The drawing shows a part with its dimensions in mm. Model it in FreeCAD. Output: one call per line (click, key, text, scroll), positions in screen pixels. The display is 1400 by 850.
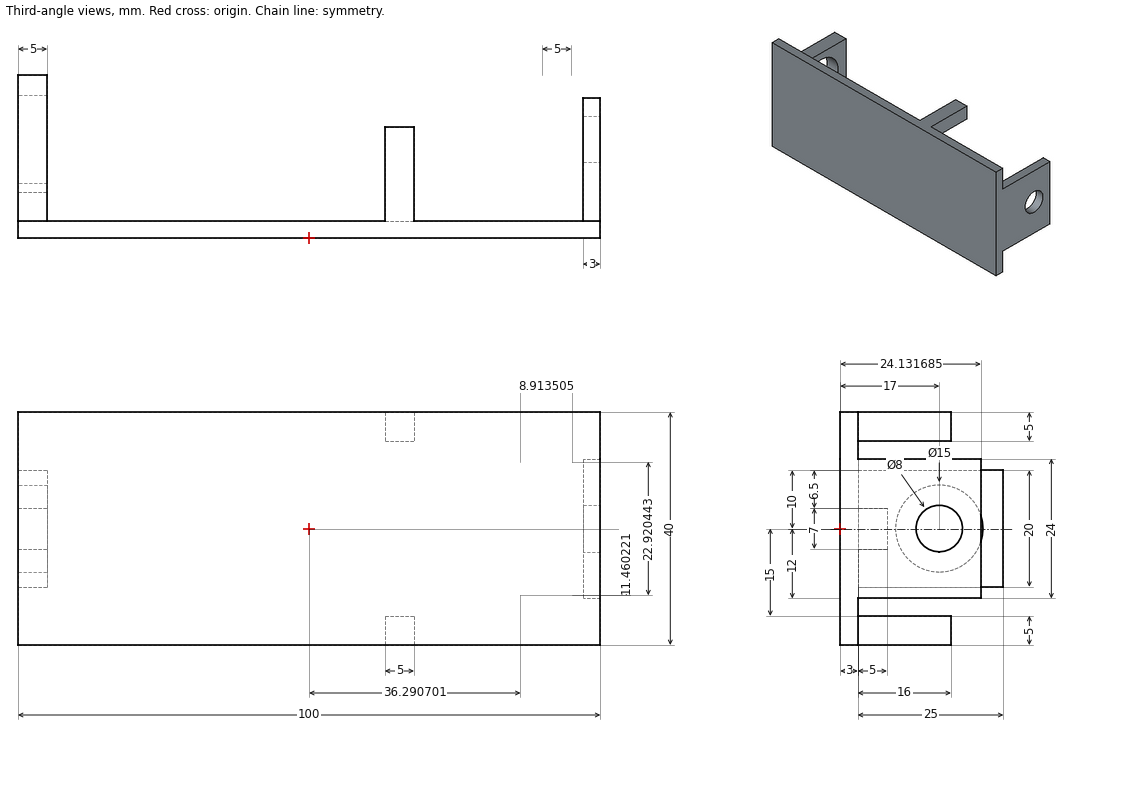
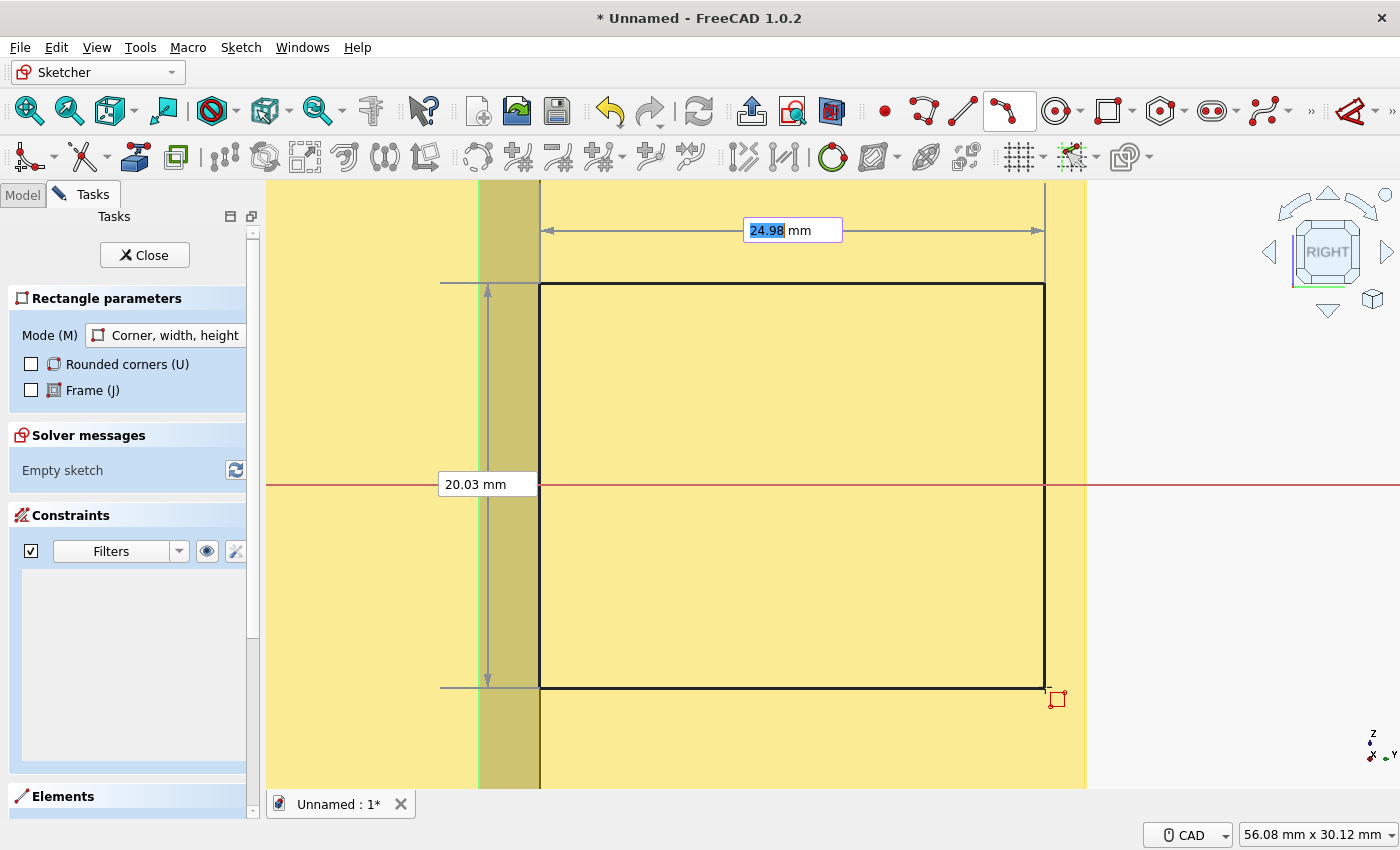
text(25)
key(Tab)
text(20)
key(Return)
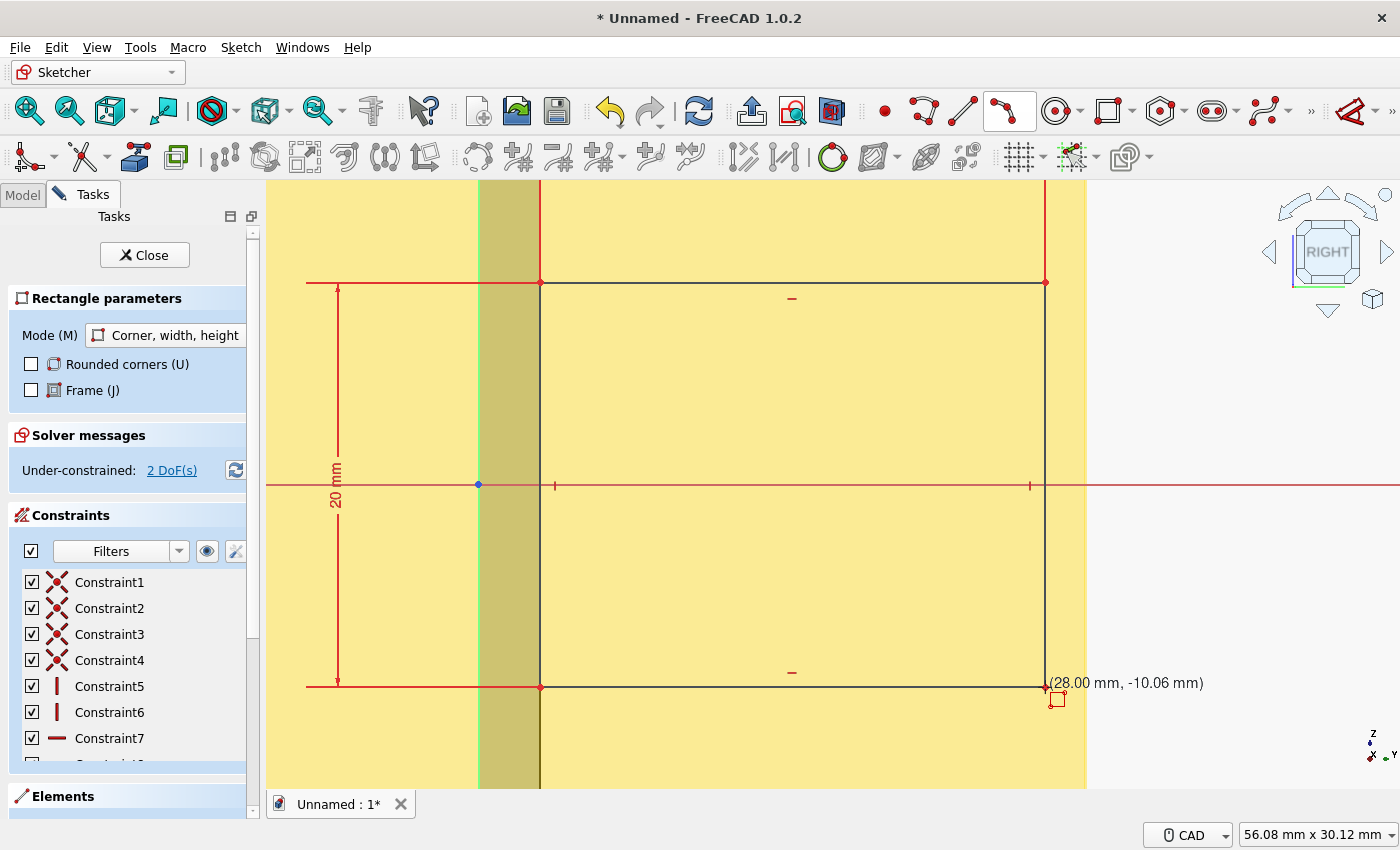
click(1056, 112)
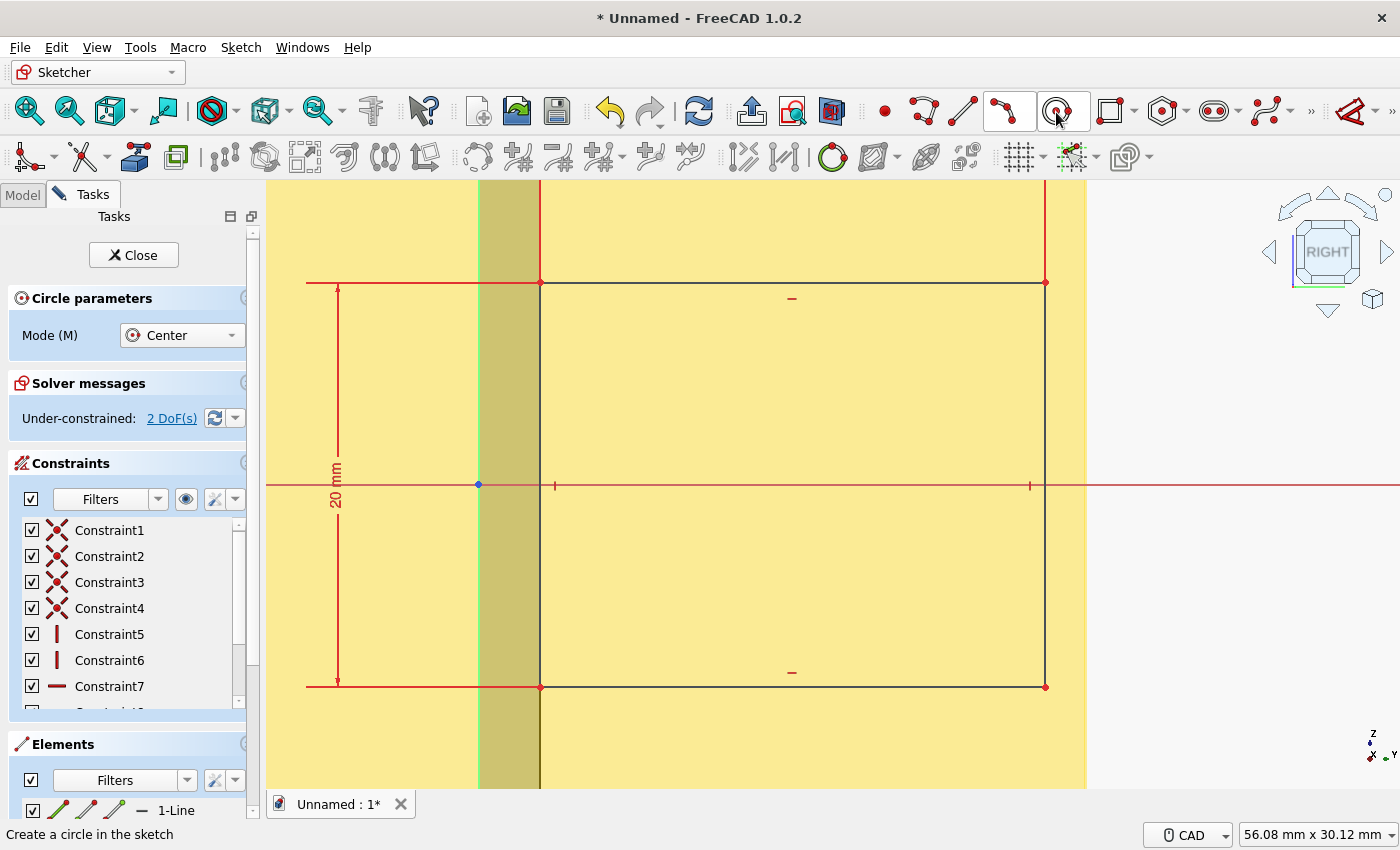
click(823, 484)
move(930, 377)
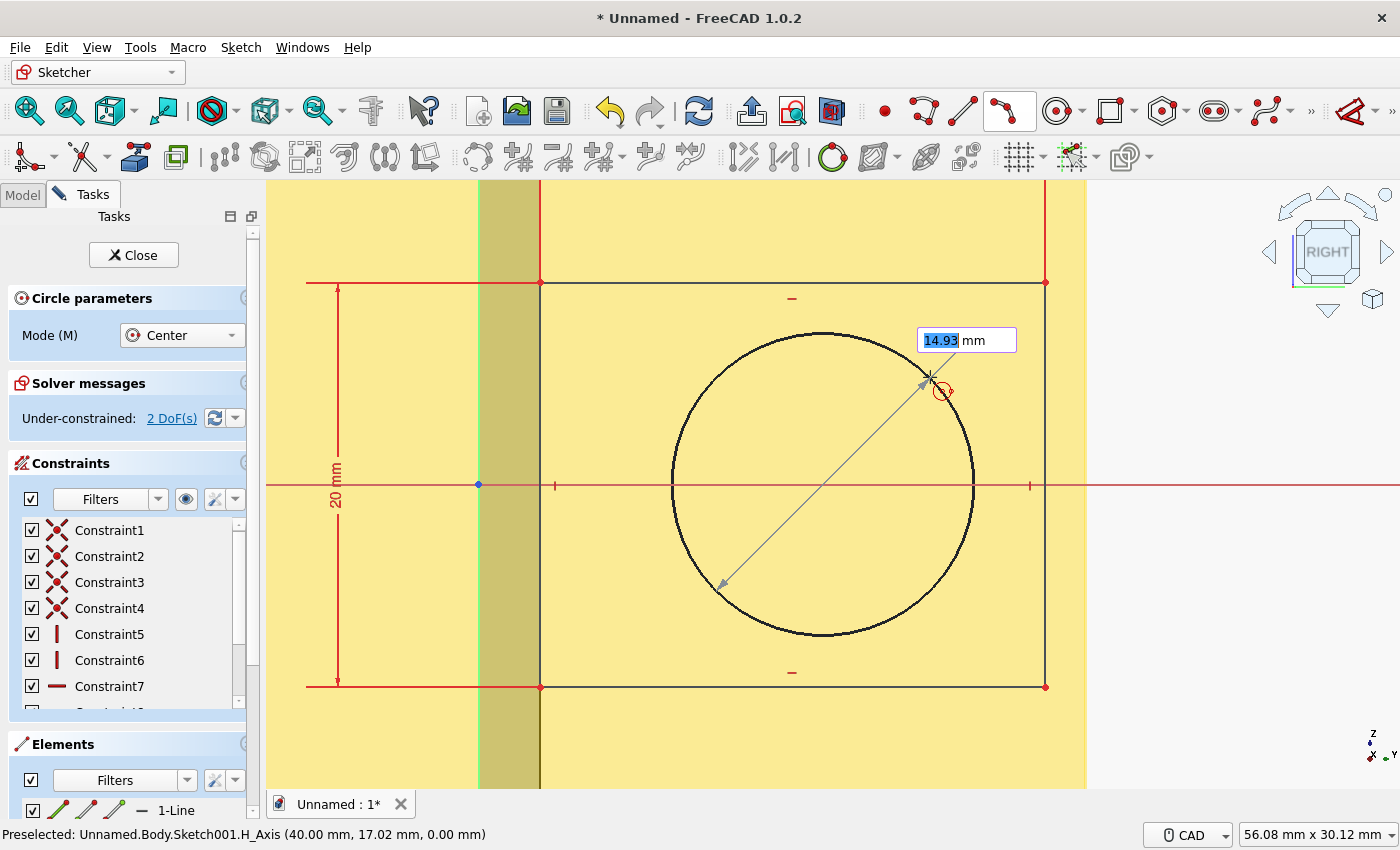
text(15)
key(Return)
key(Escape)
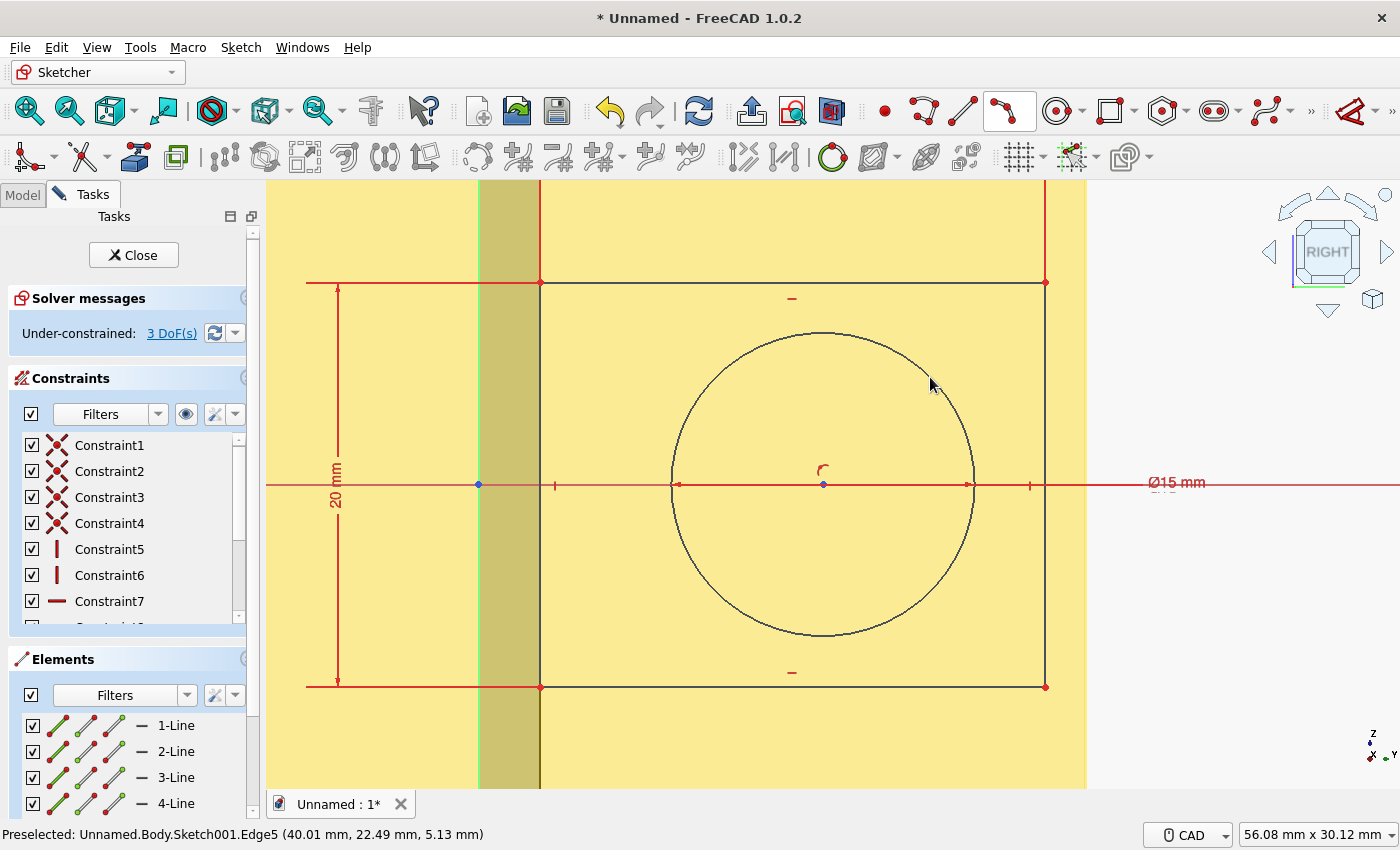
click(1350, 112)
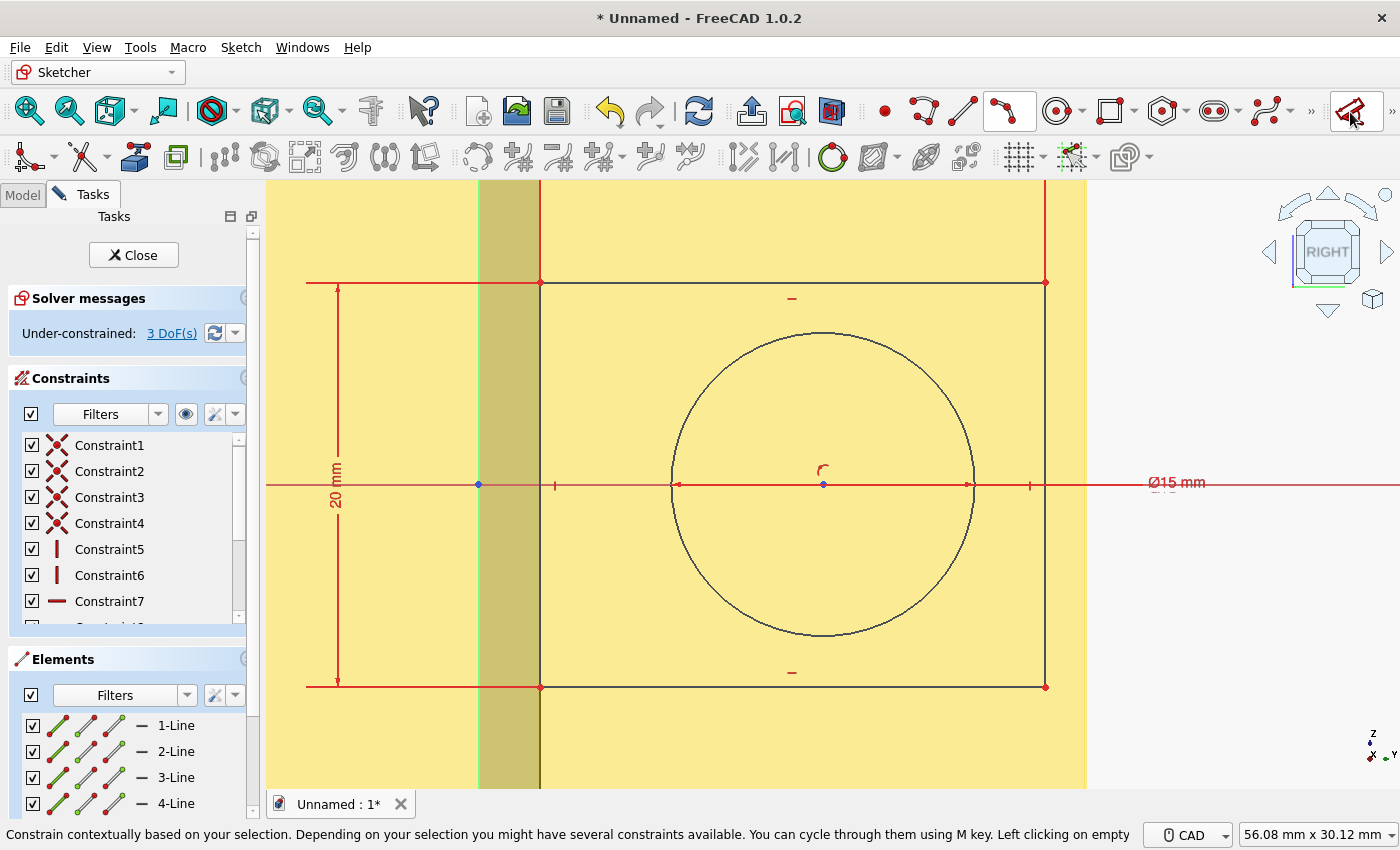
click(540, 283)
click(509, 249)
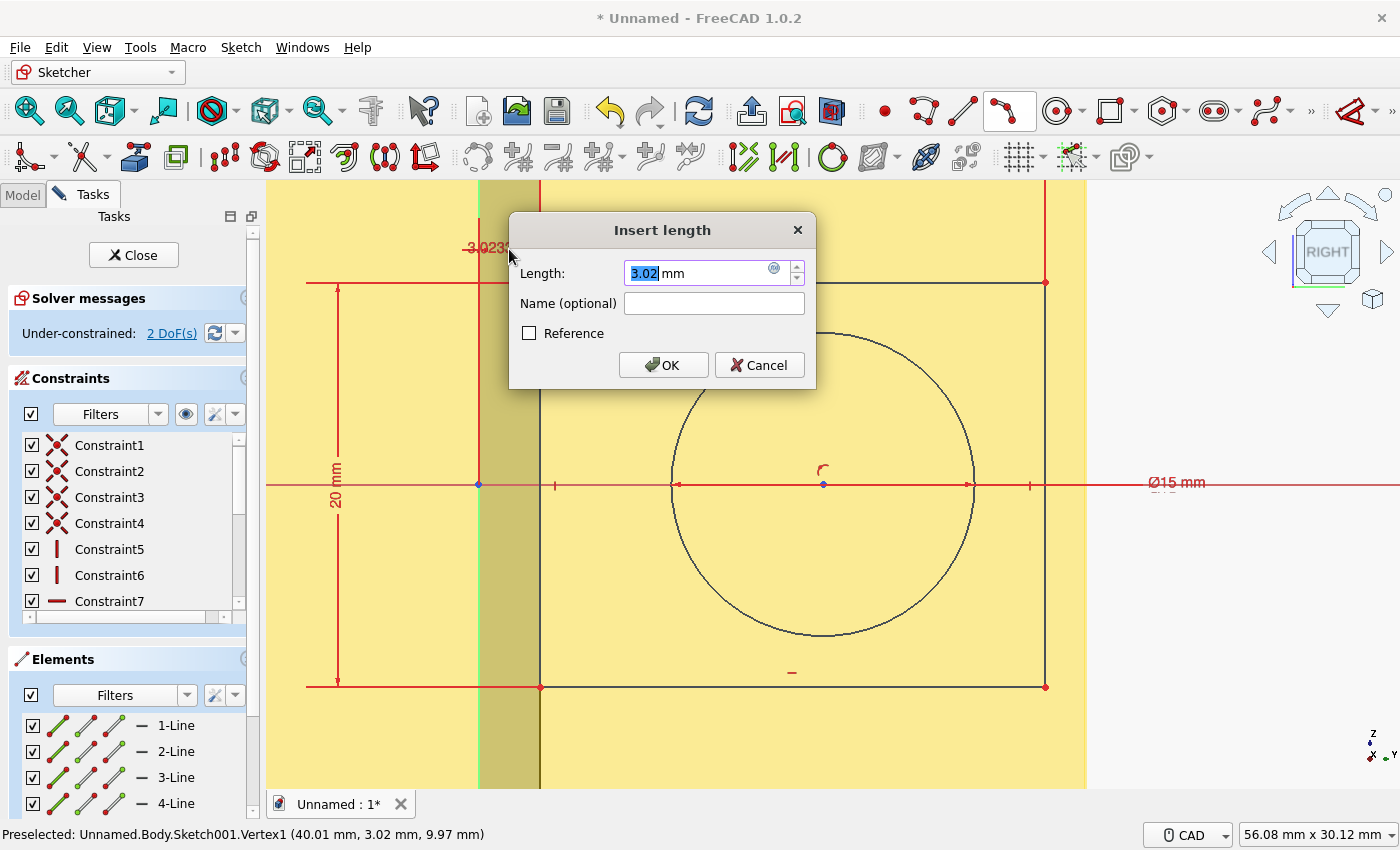
text(3)
key(Return)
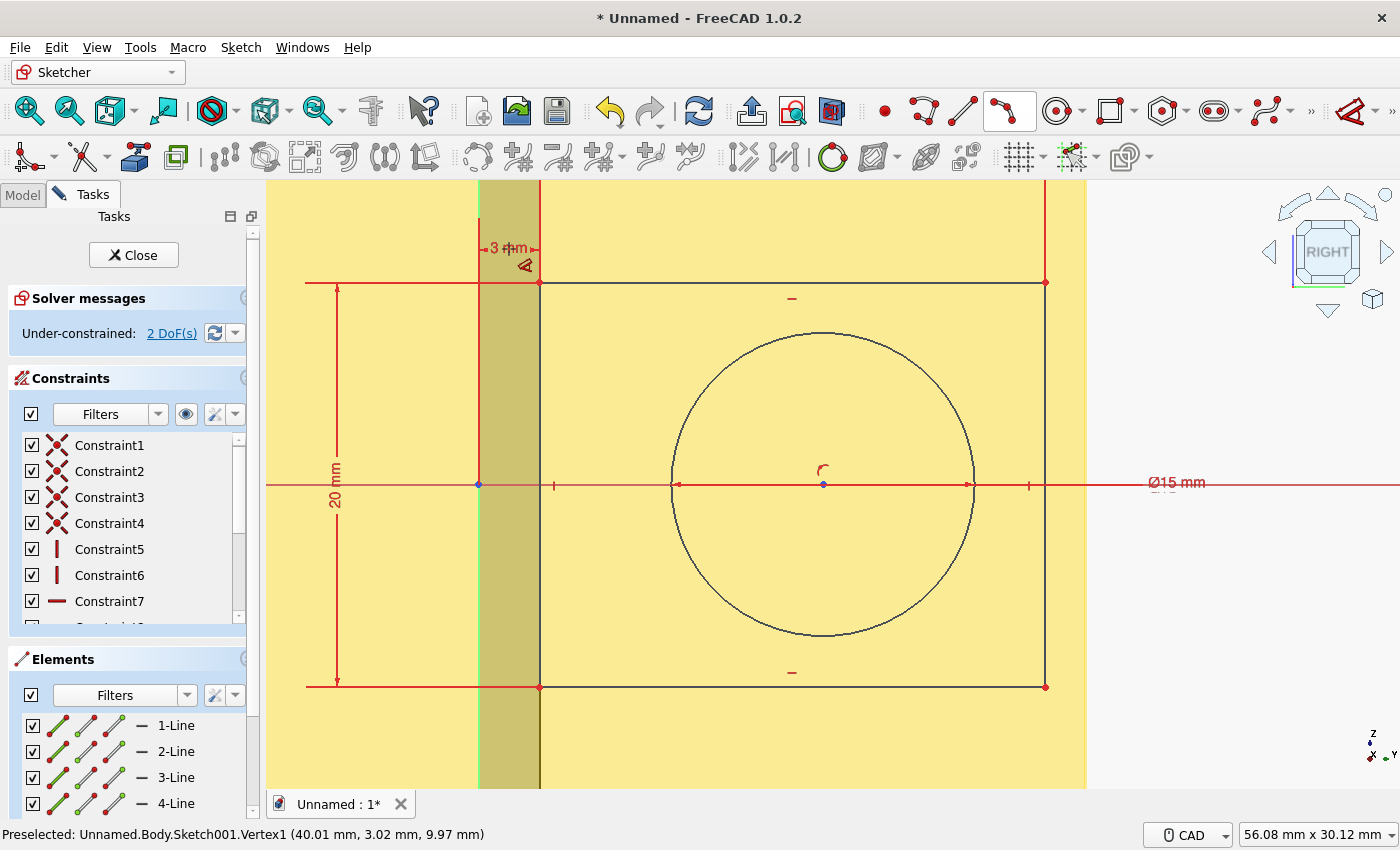
click(823, 484)
click(651, 518)